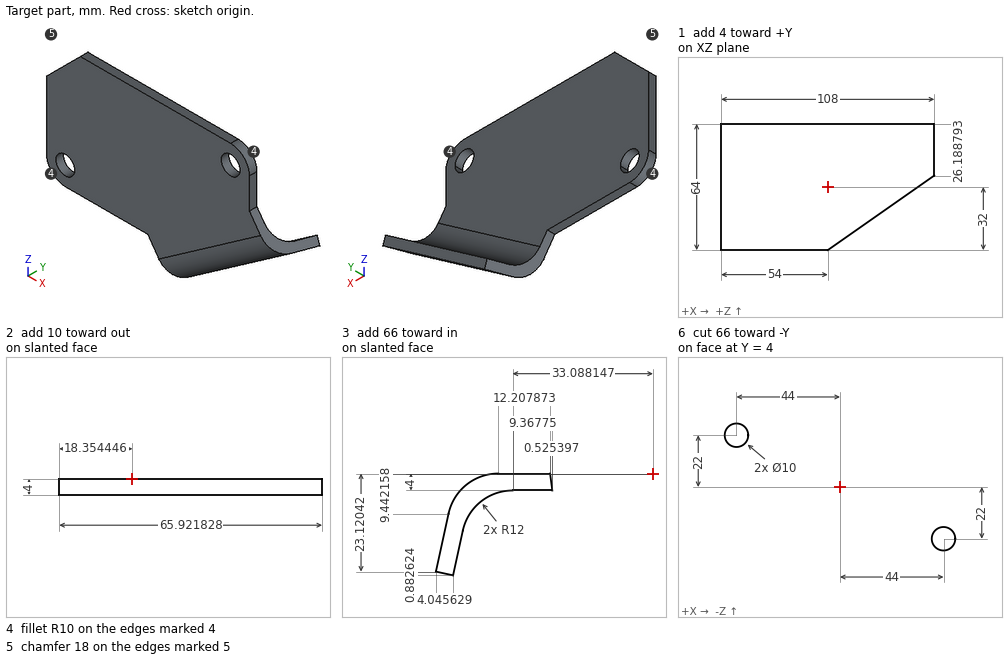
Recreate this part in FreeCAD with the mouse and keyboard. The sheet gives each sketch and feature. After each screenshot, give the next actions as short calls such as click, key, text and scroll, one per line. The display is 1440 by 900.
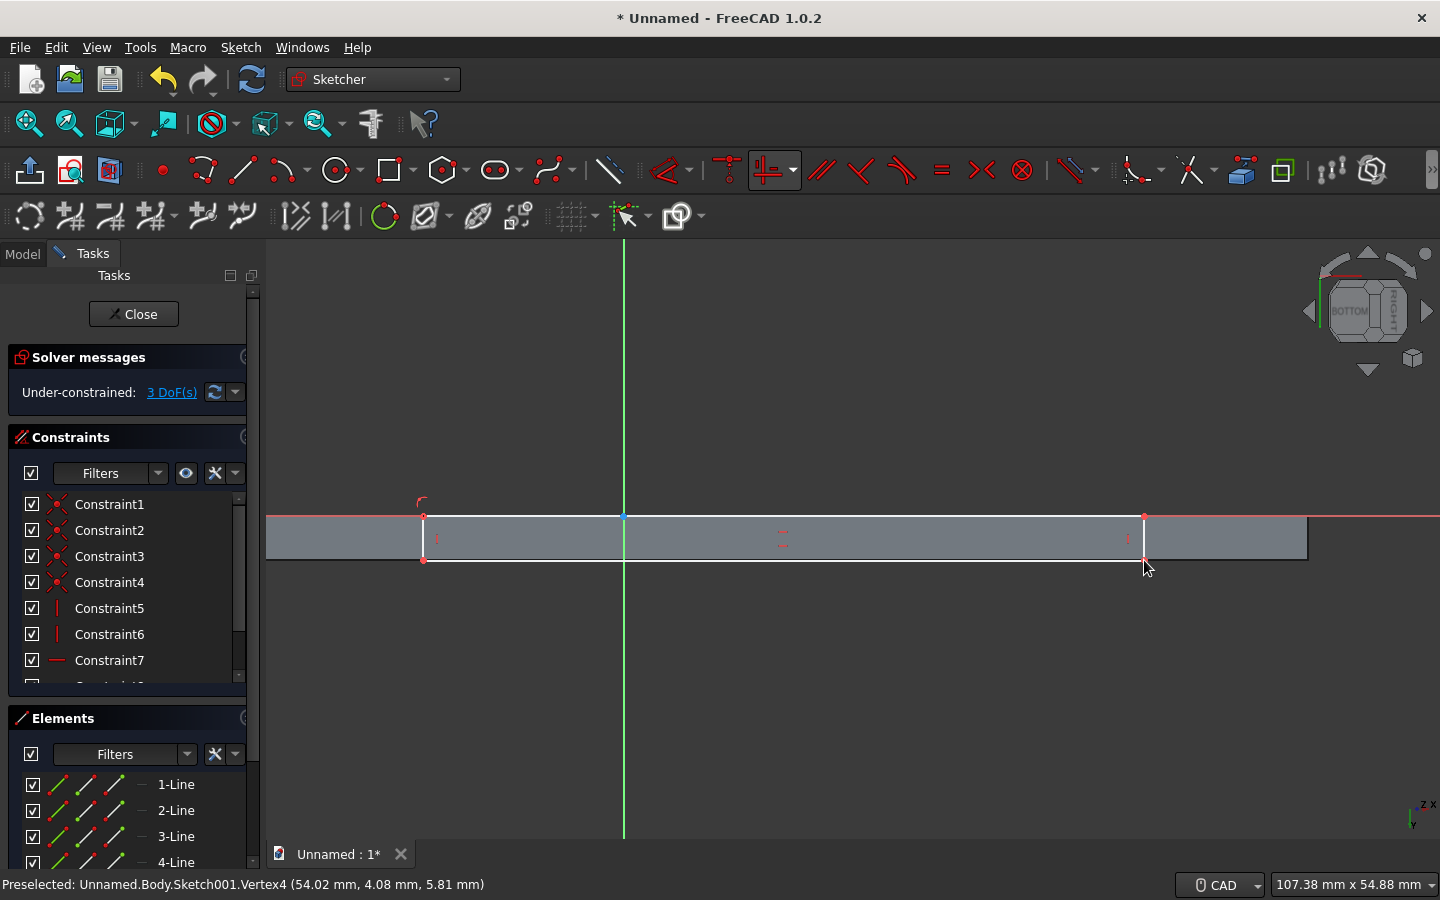
click(423, 530)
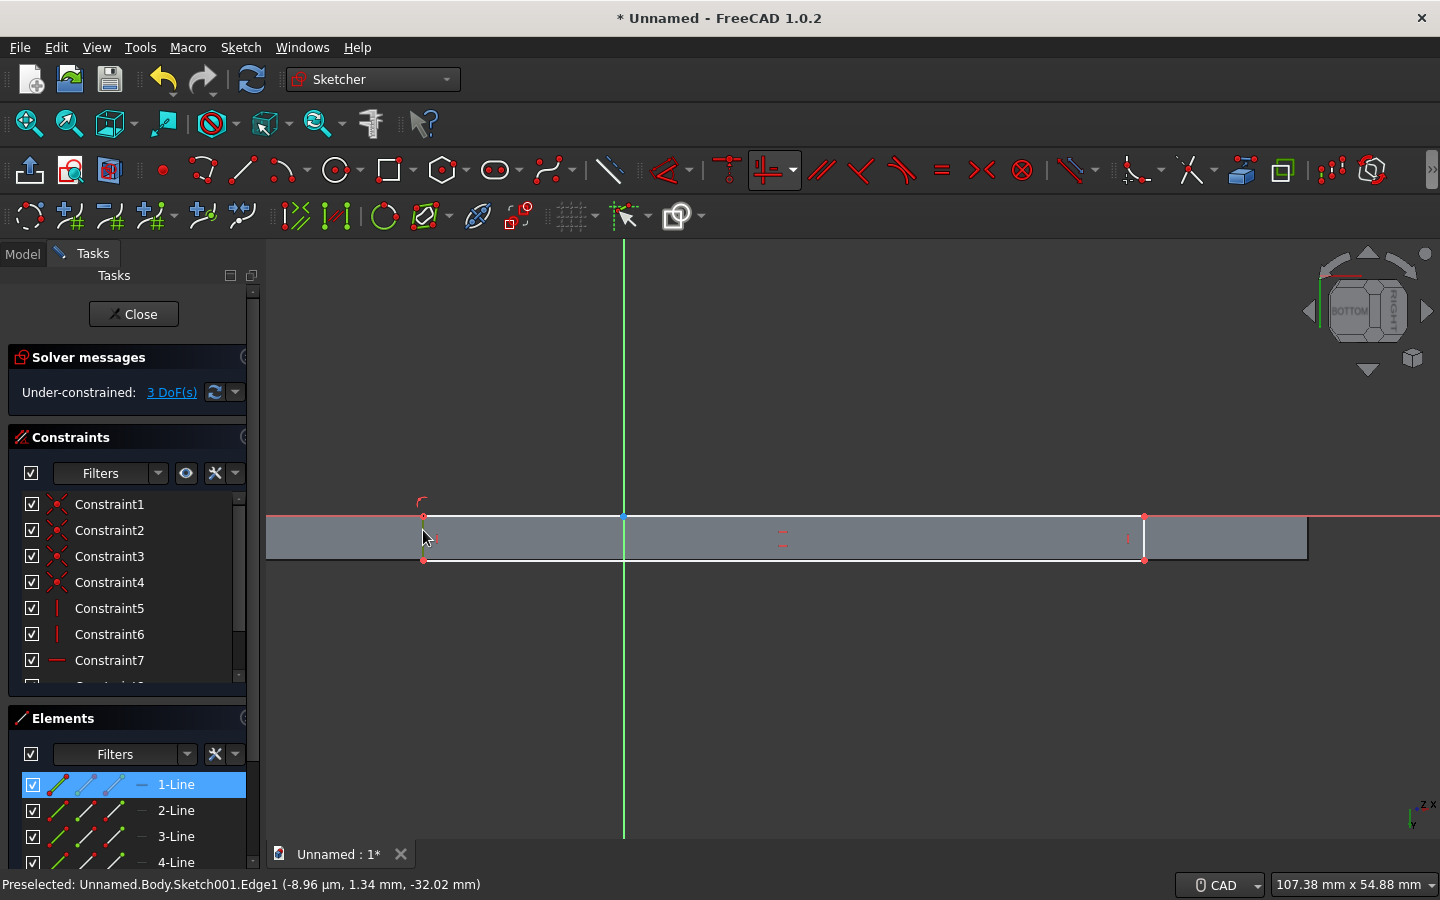
key(i)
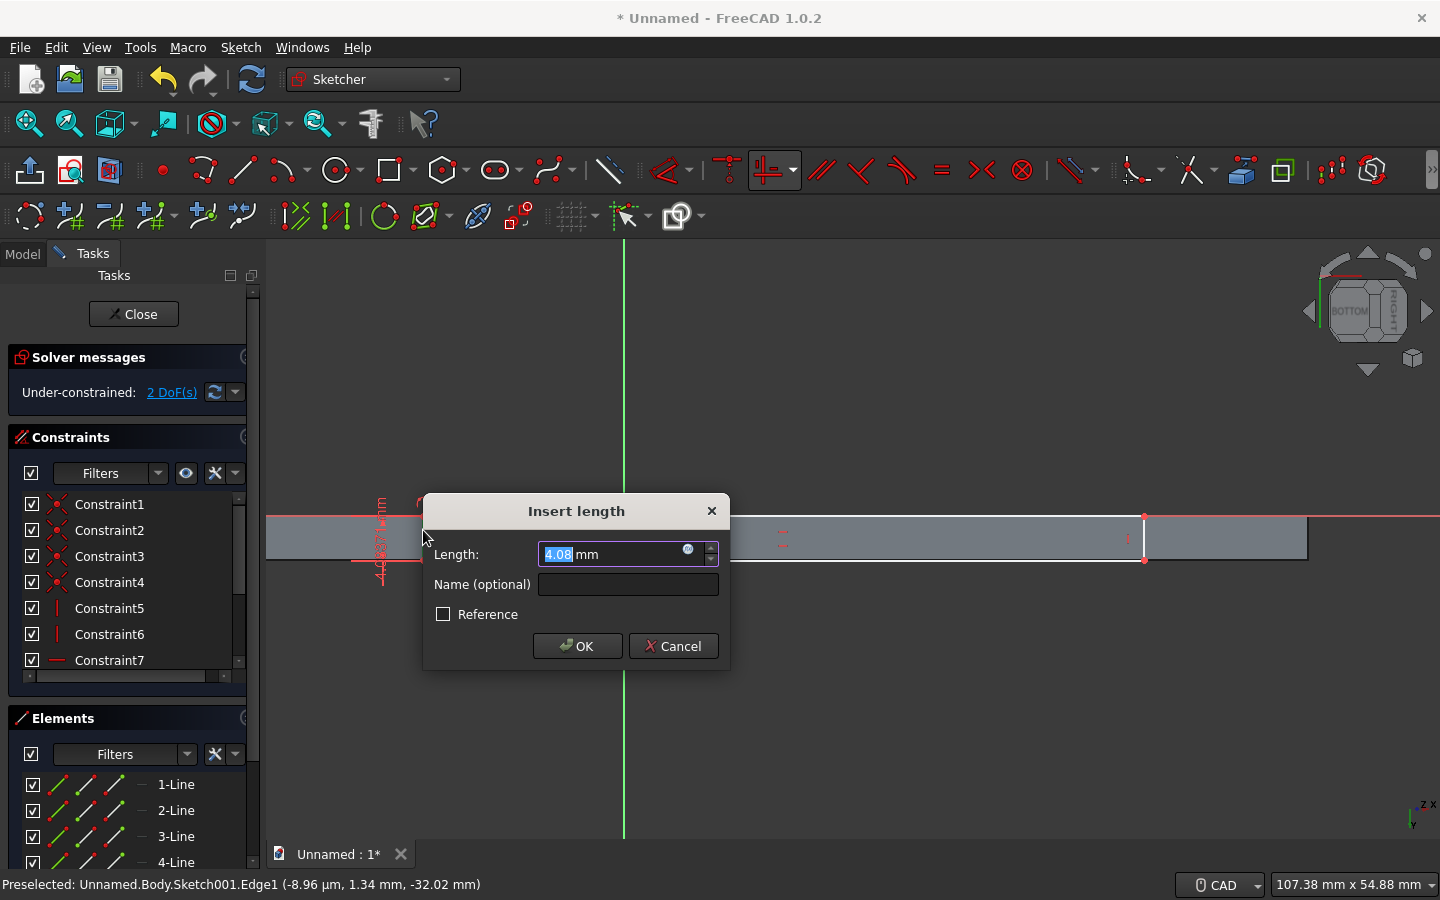
text(4)
key(Return)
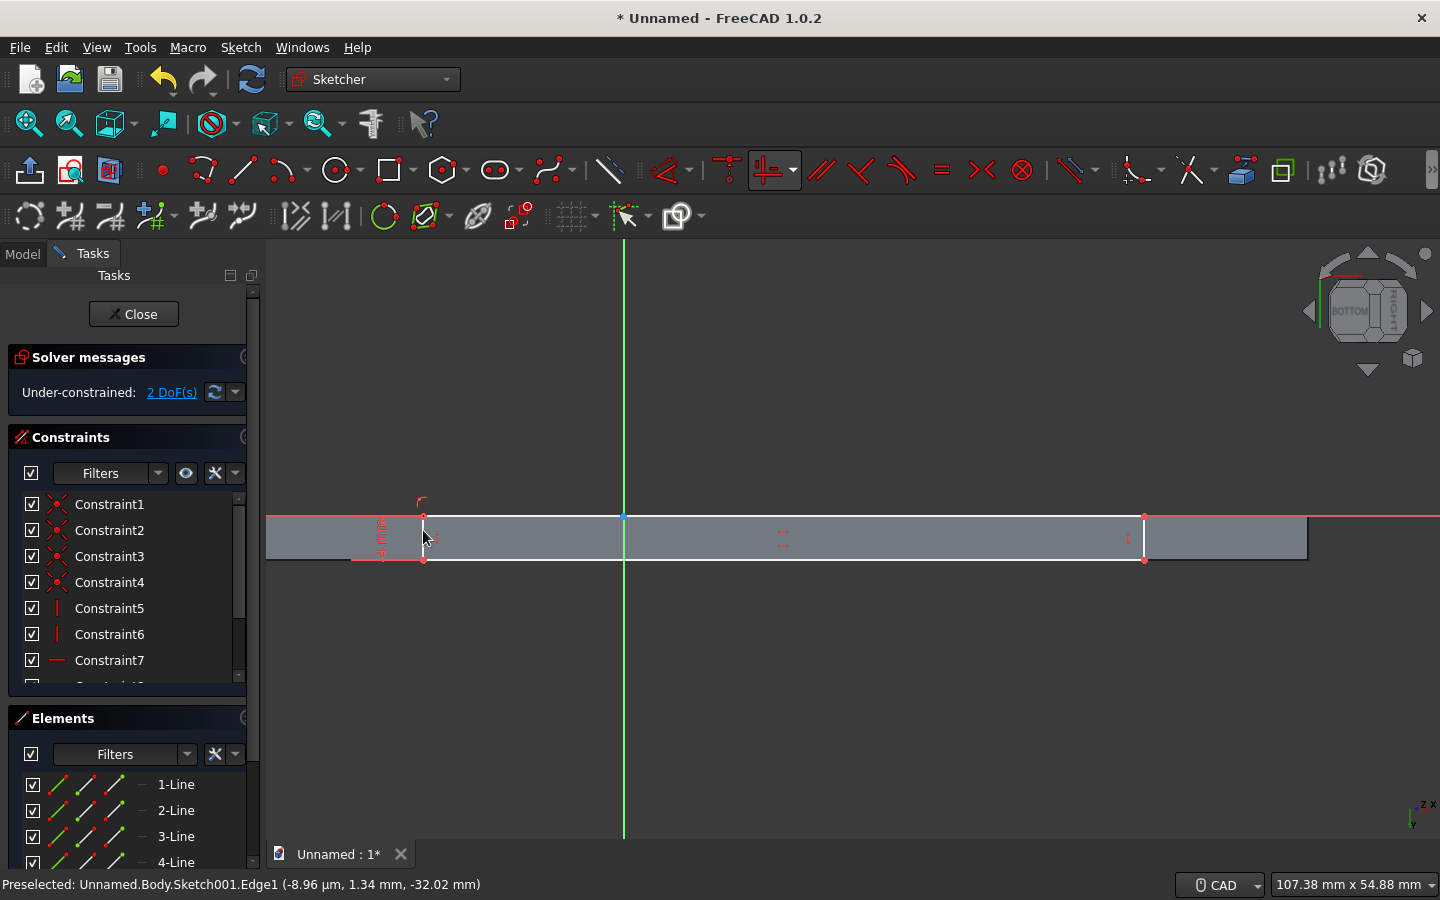
click(639, 560)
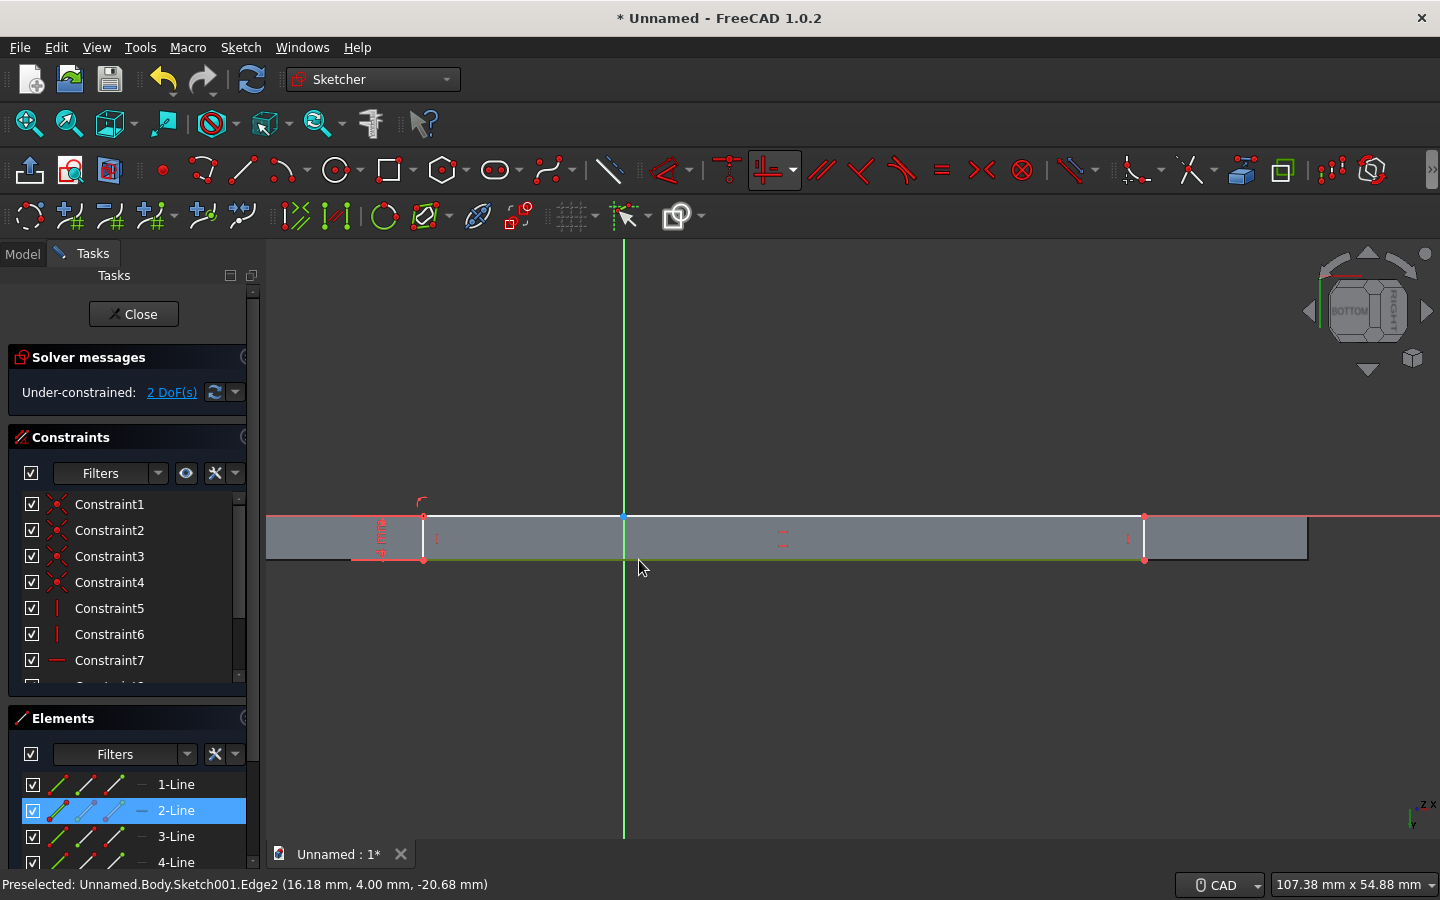
key(l)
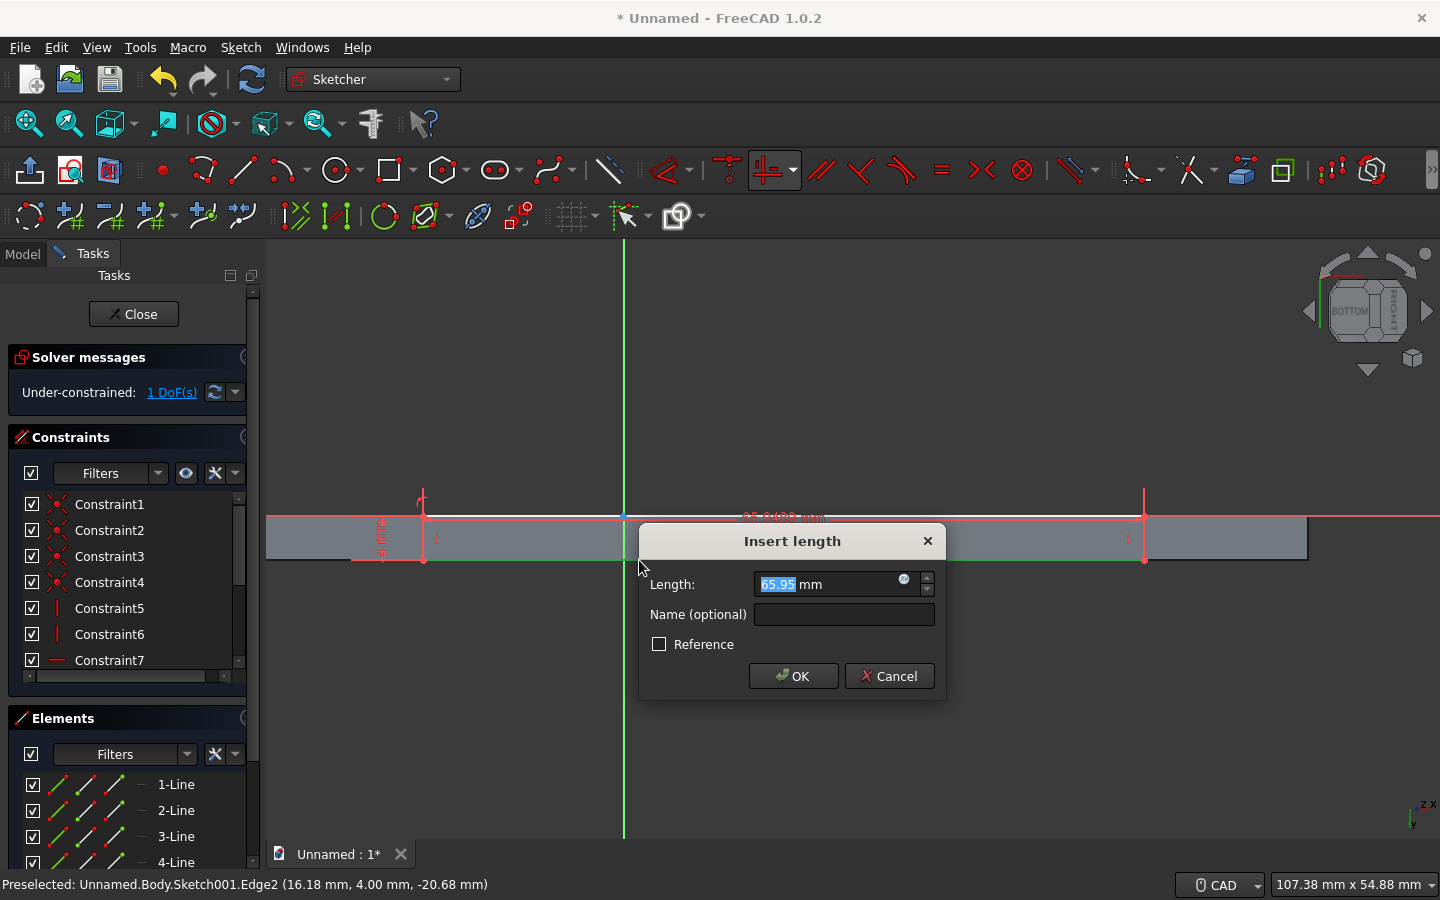
text(65.921828)
key(Return)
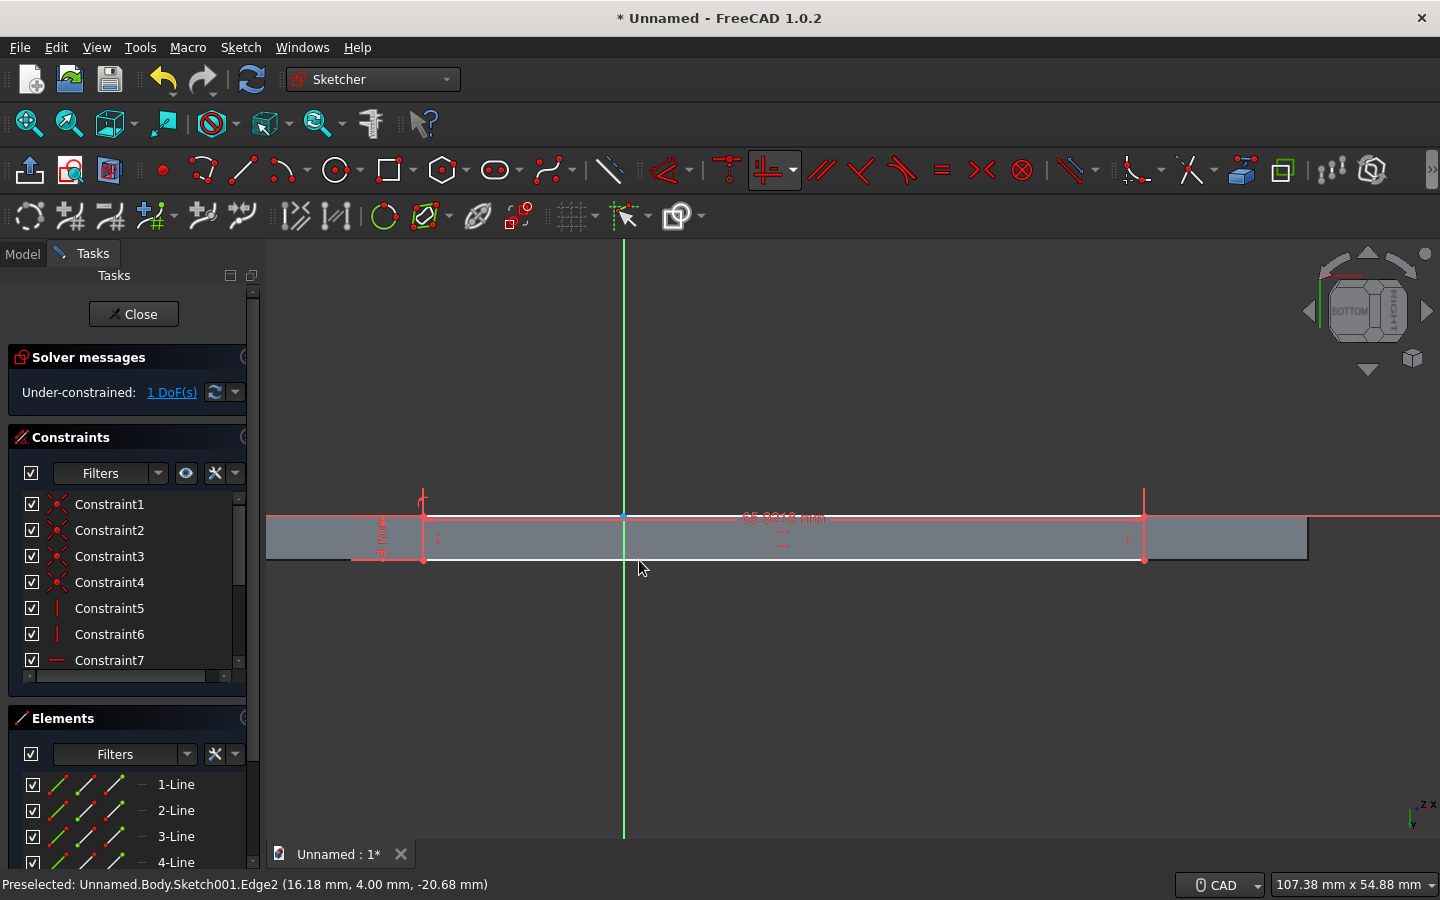
click(423, 516)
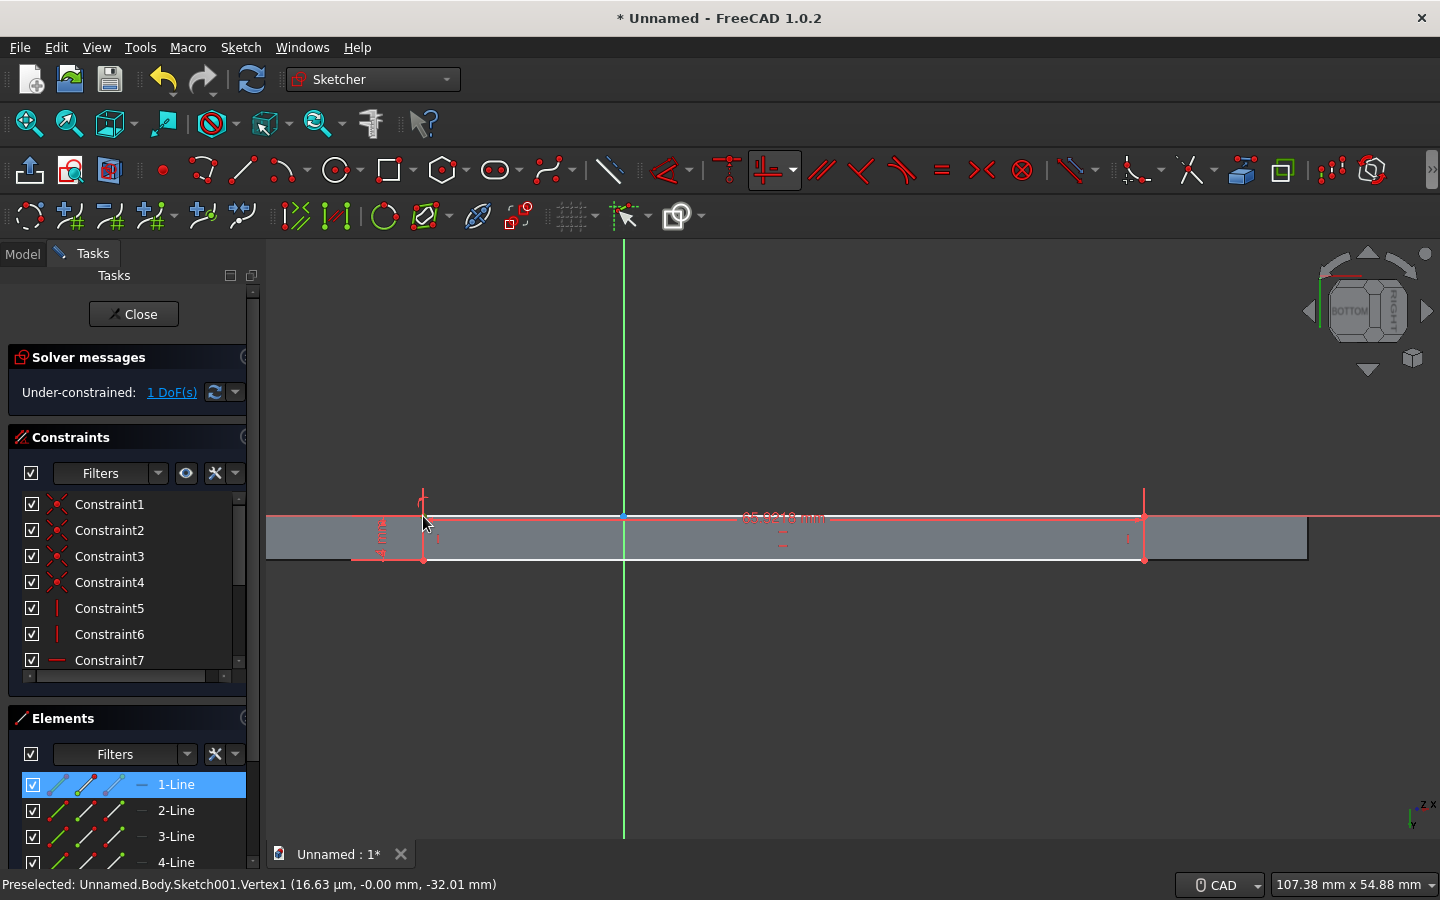
key(l)